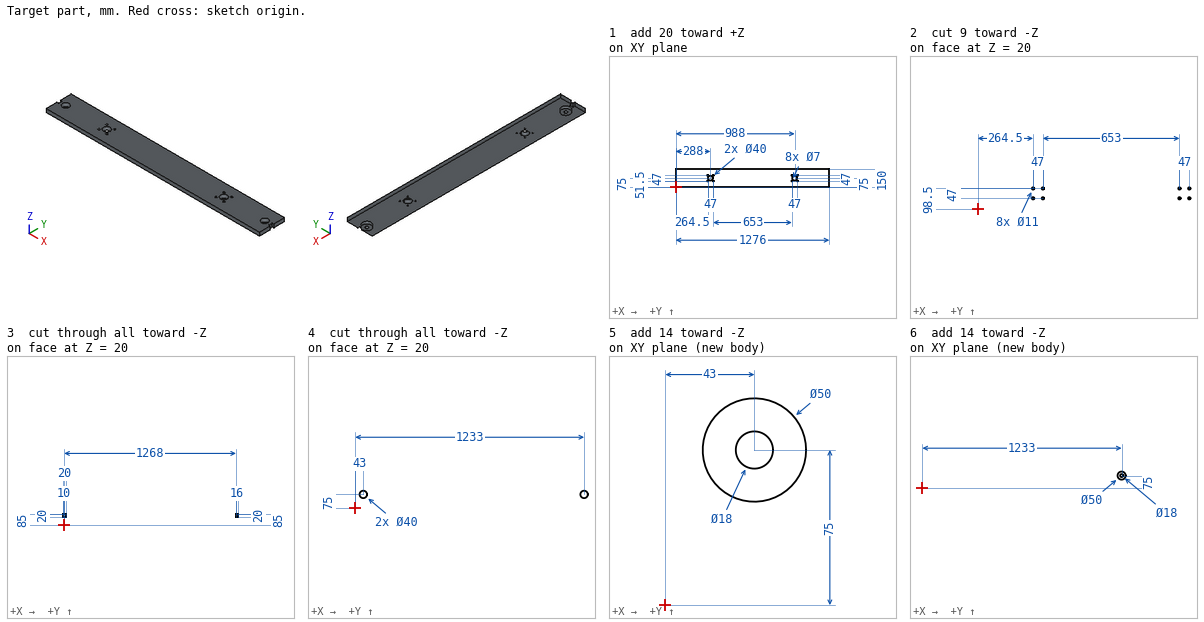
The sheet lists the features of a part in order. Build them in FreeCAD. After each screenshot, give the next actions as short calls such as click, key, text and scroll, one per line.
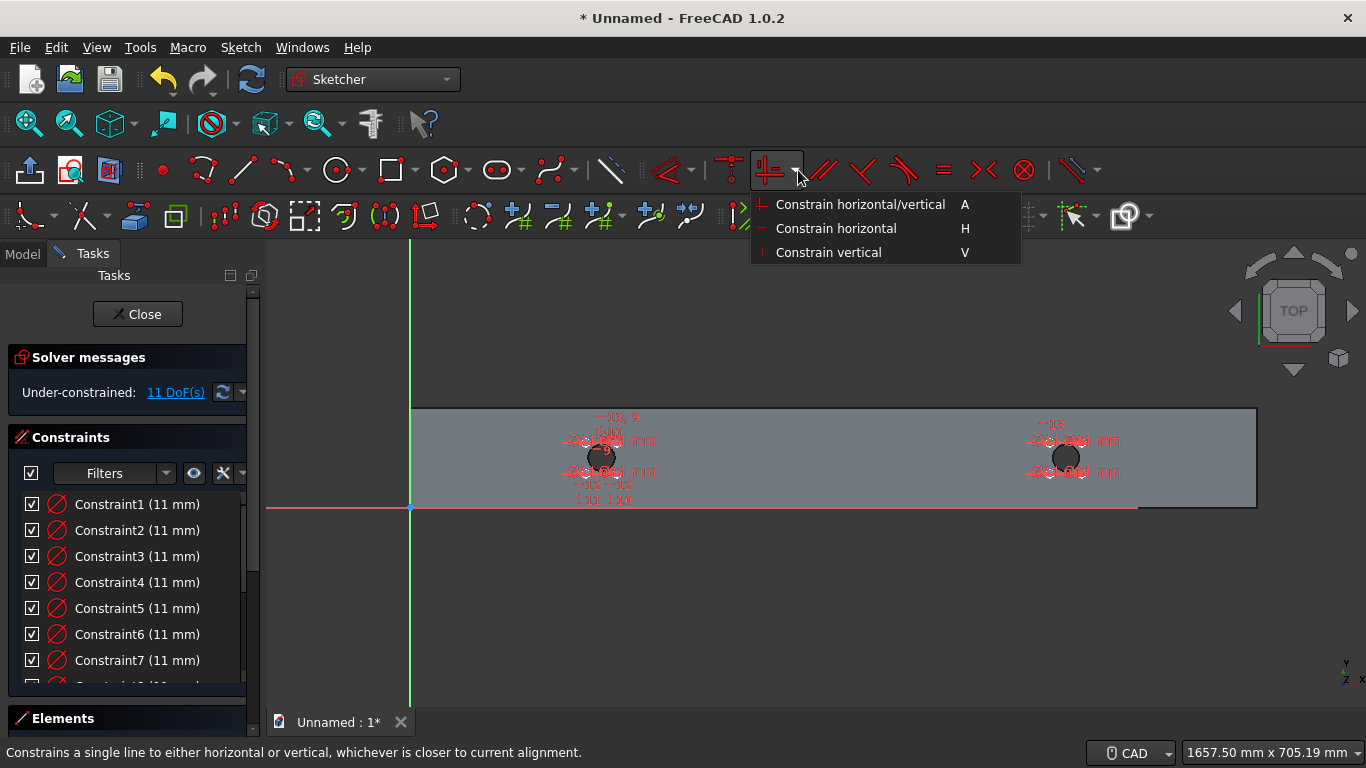
click(886, 228)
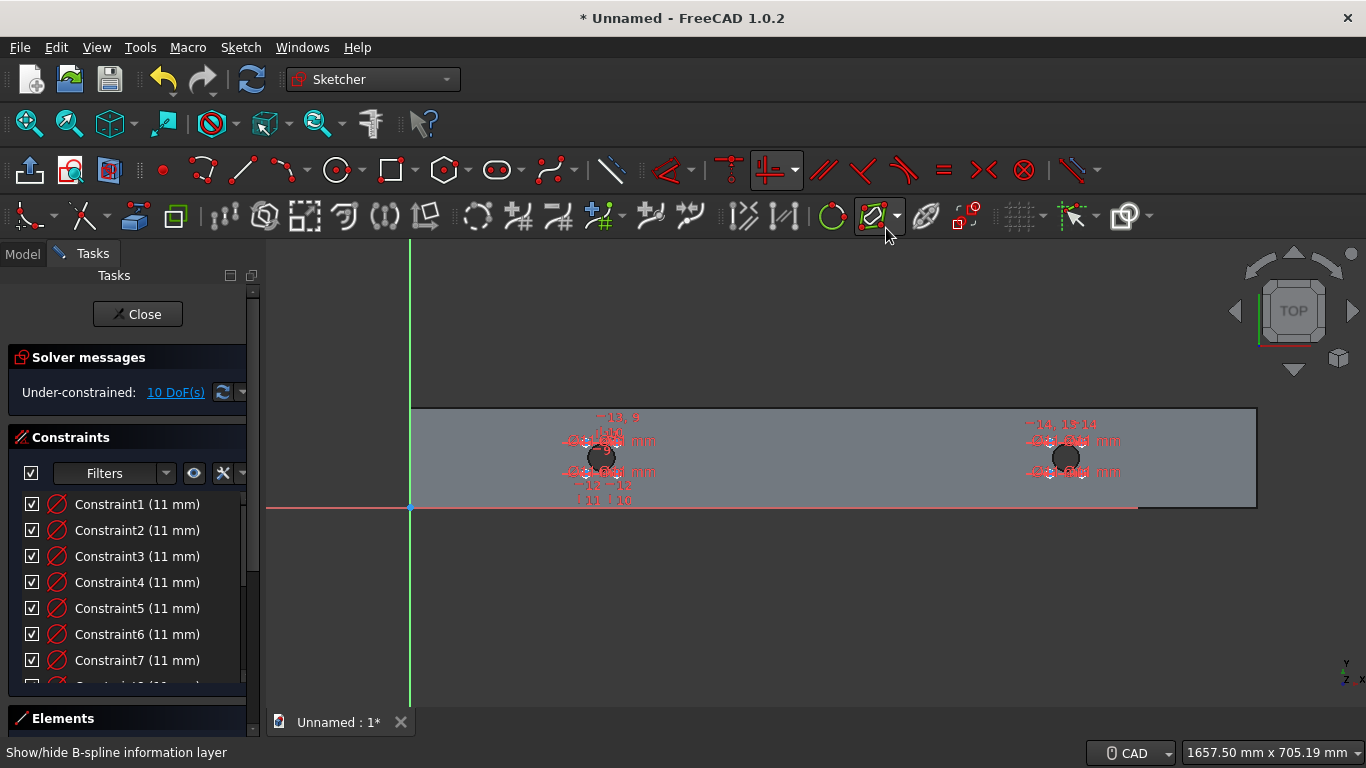
click(1082, 443)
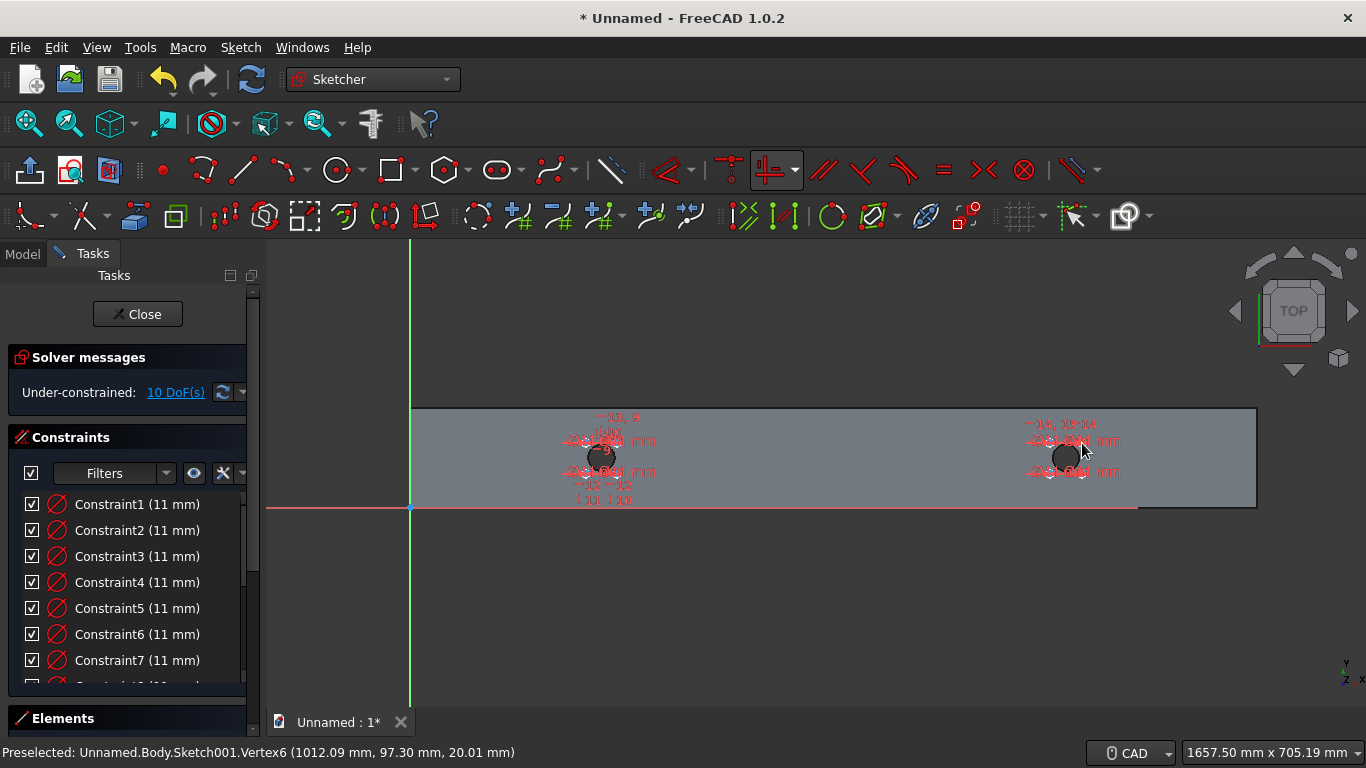
click(1082, 474)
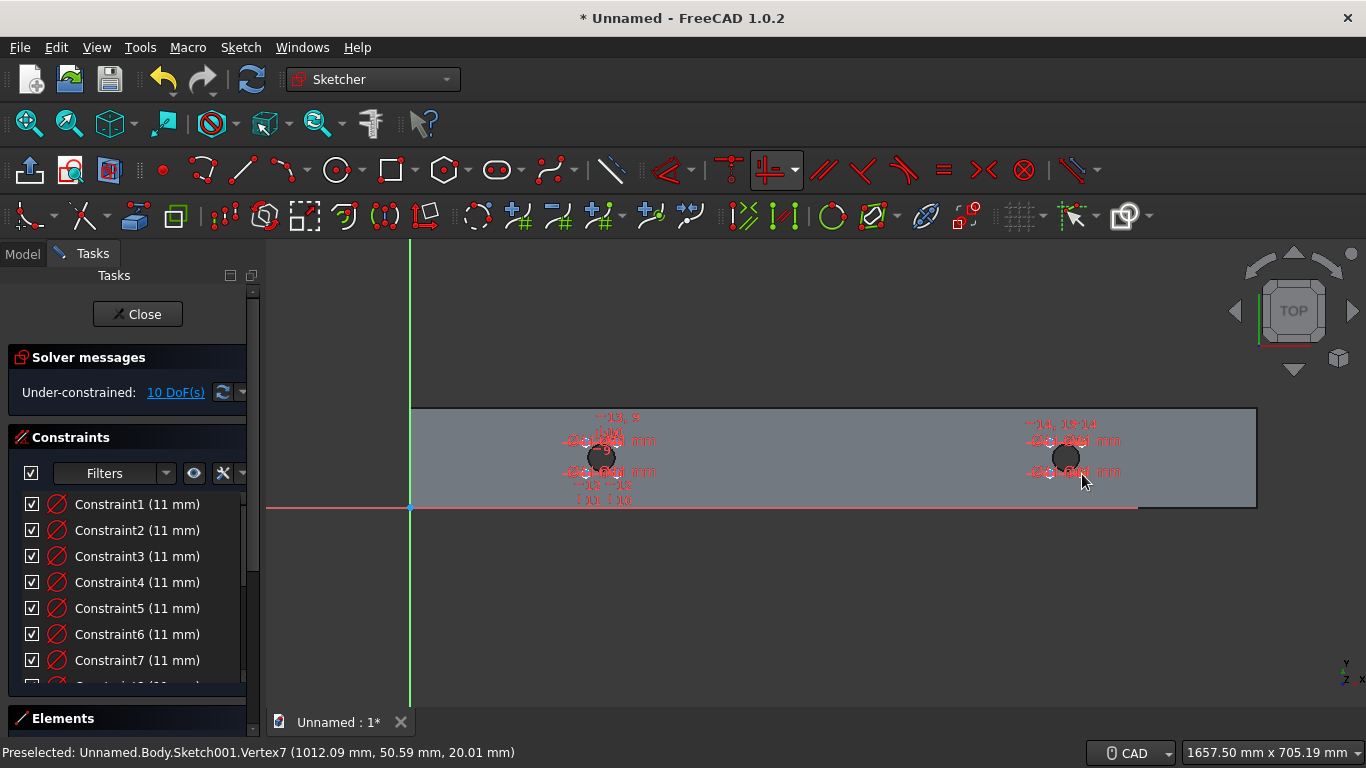
click(798, 170)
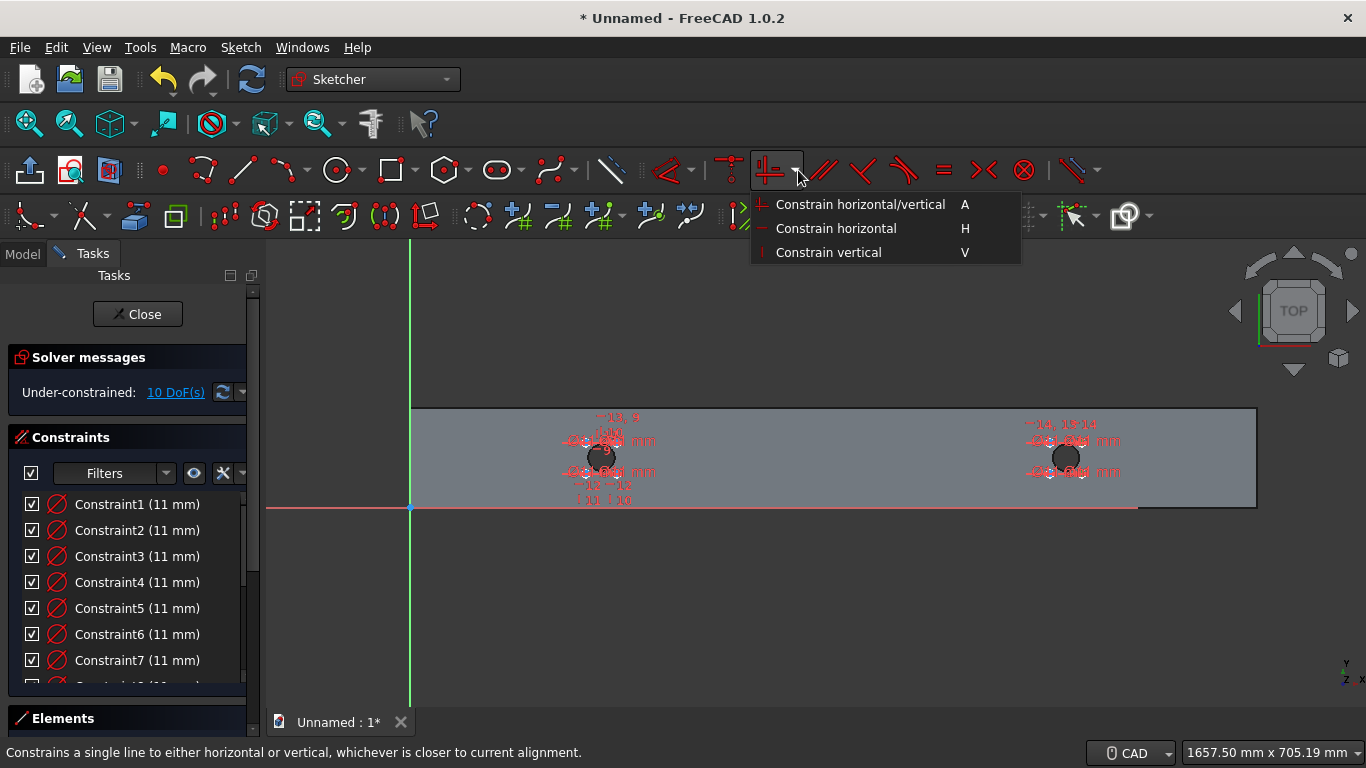
click(886, 252)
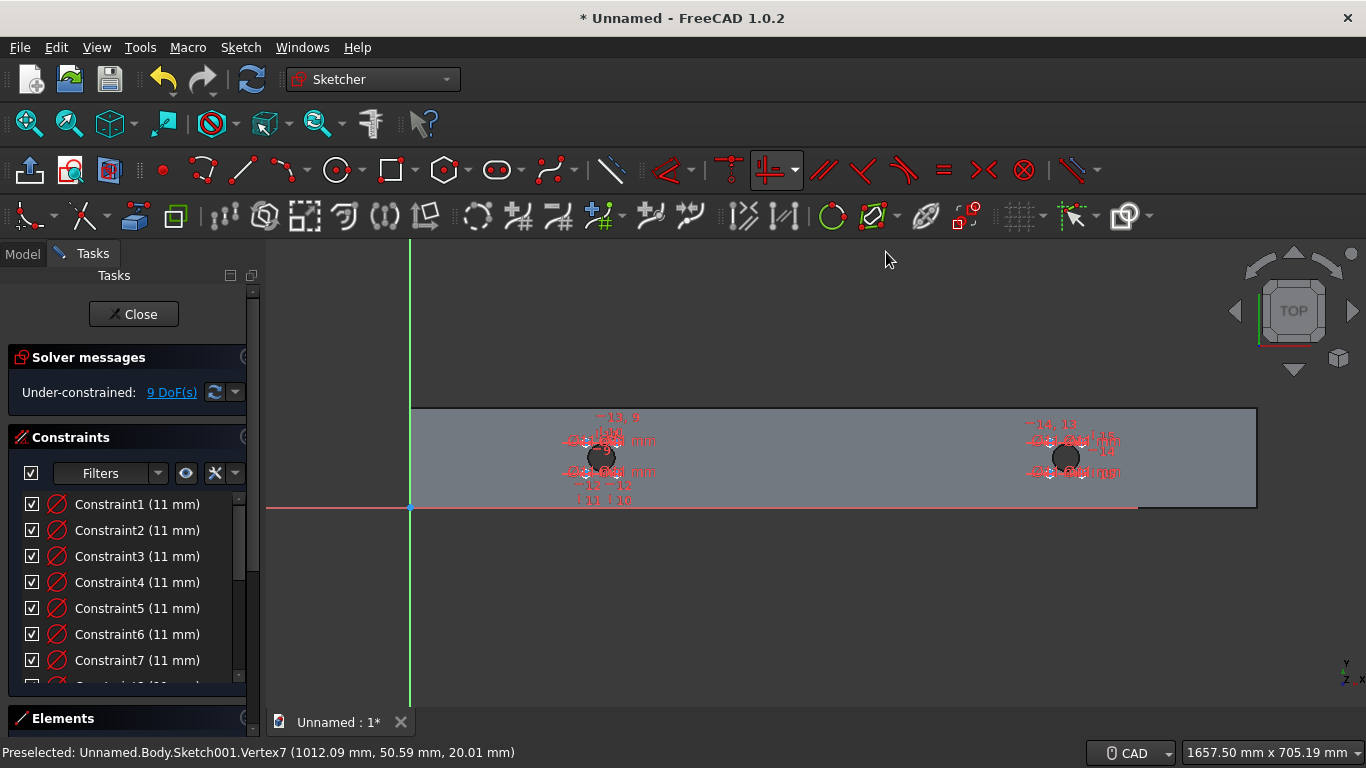
click(617, 474)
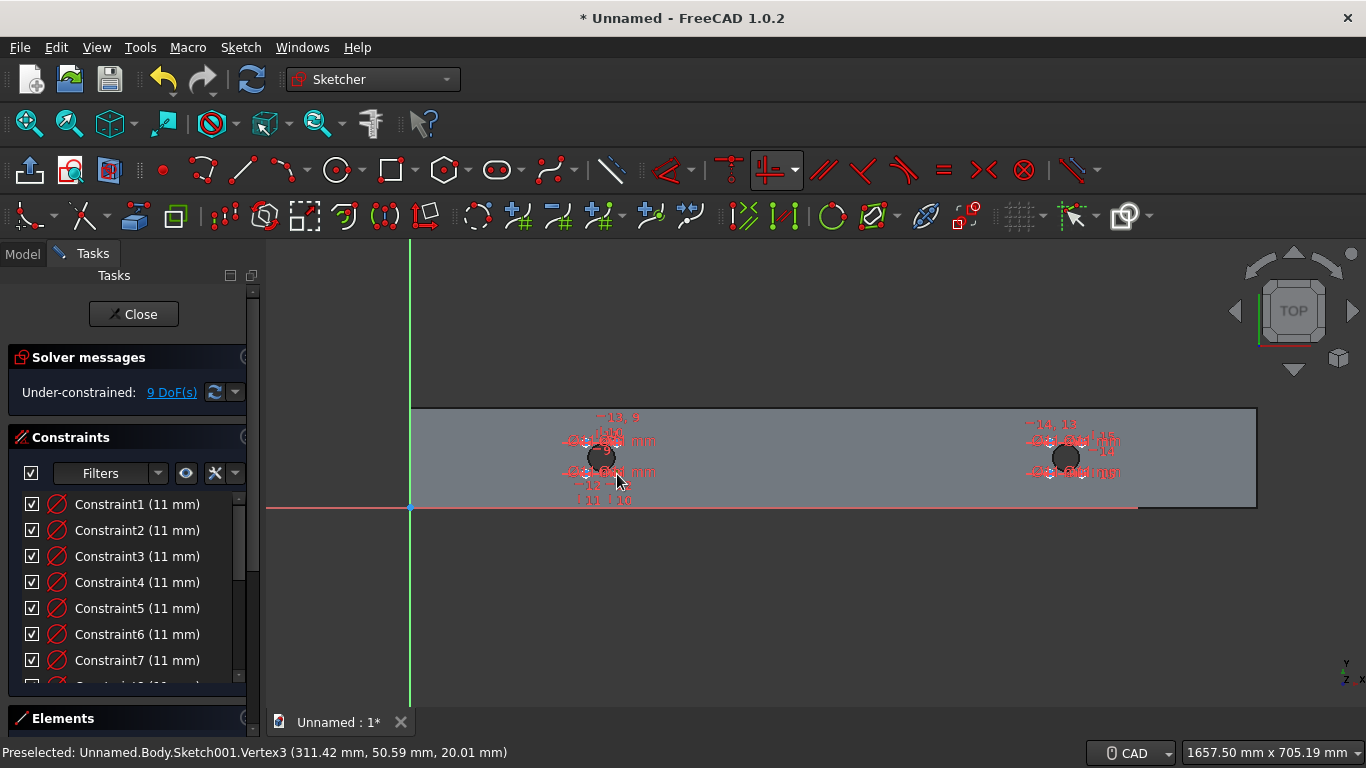
click(1082, 474)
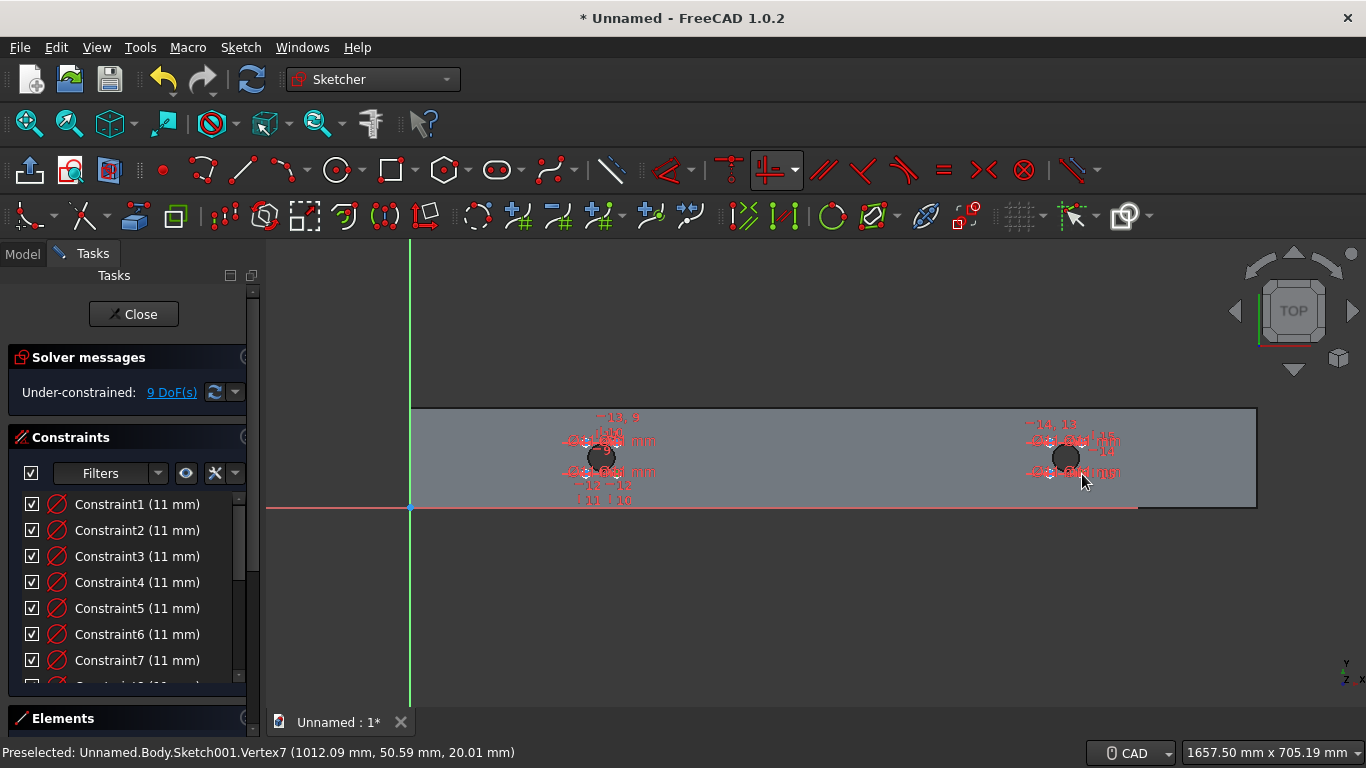
click(798, 170)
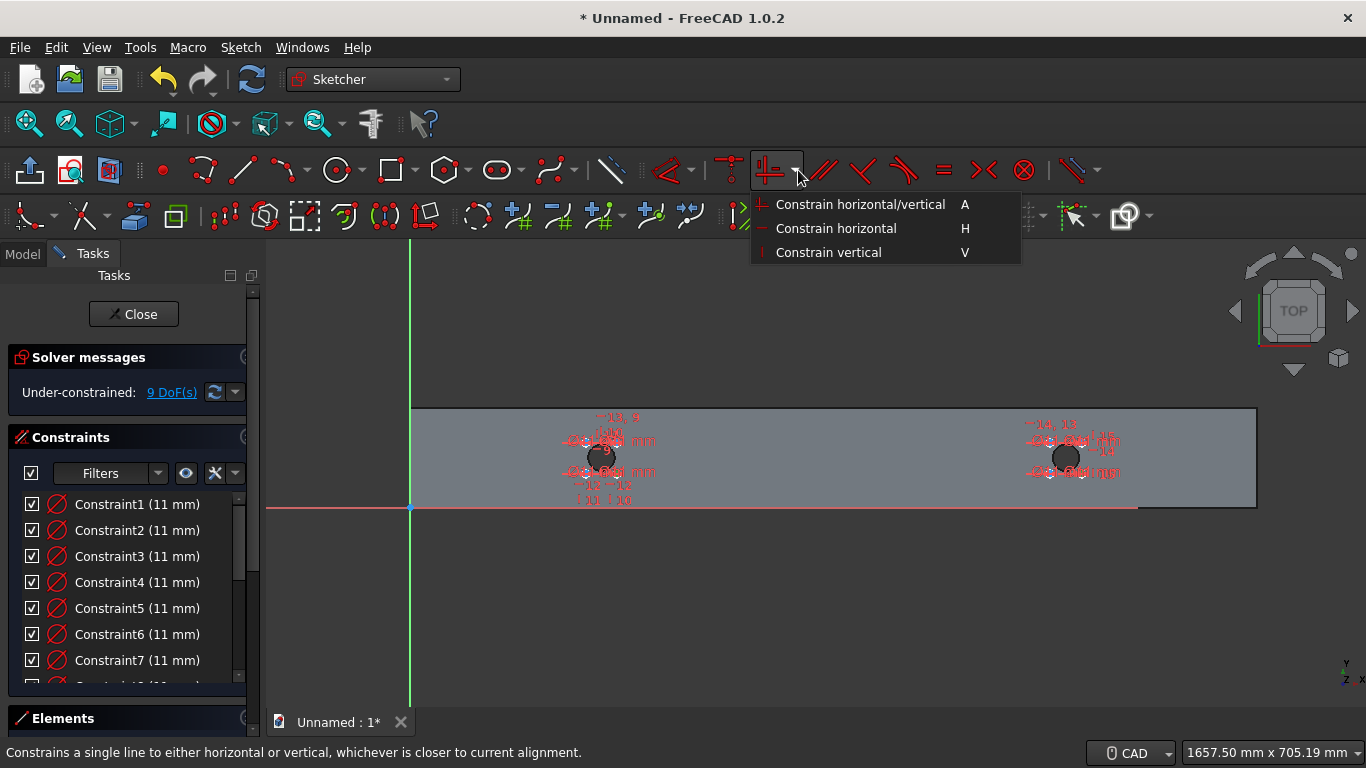
click(886, 228)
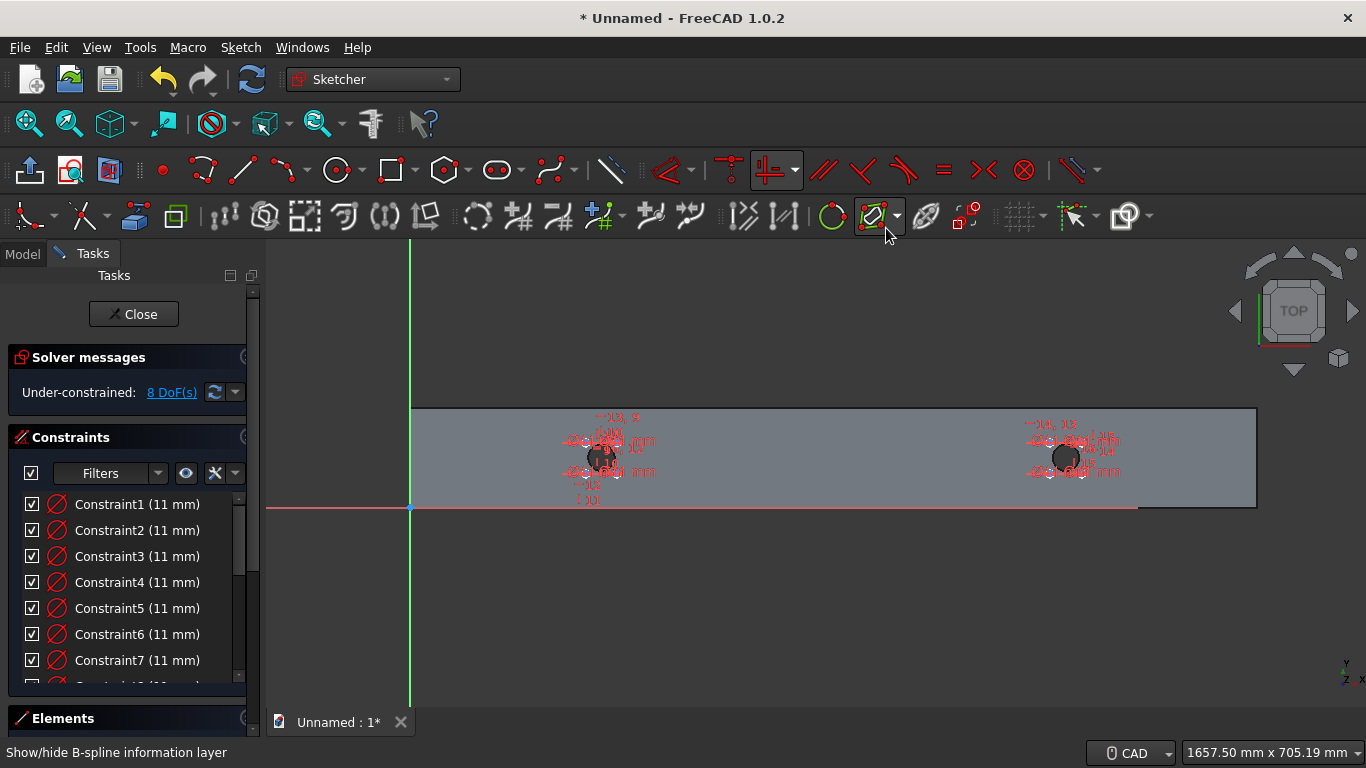
click(1050, 443)